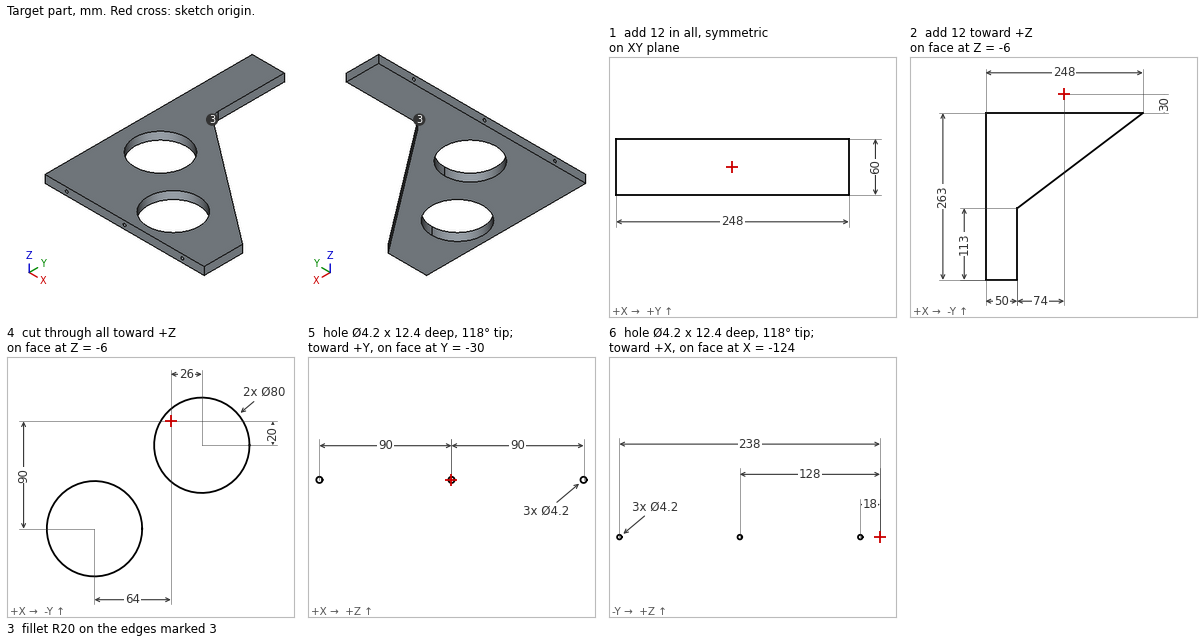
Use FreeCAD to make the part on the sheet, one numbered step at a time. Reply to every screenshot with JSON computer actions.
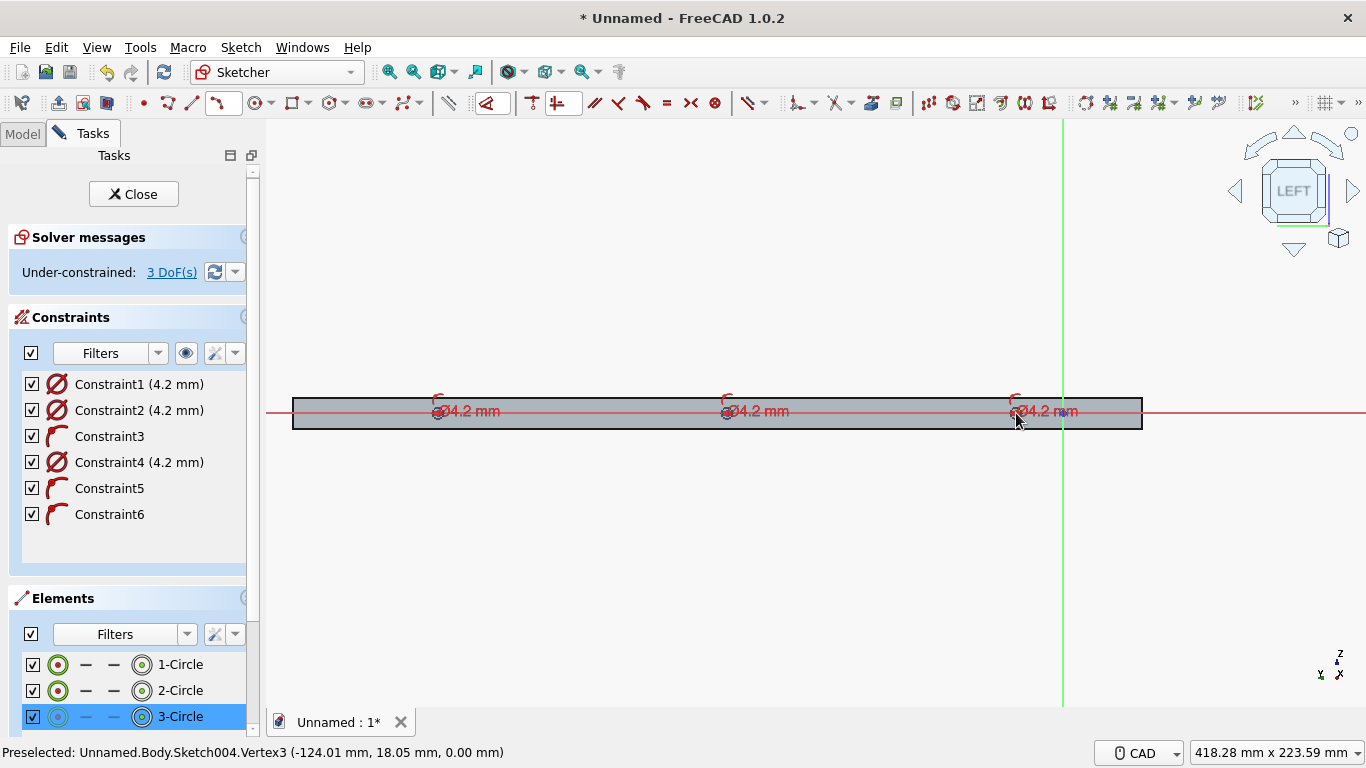
{"action": "key", "text": "l"}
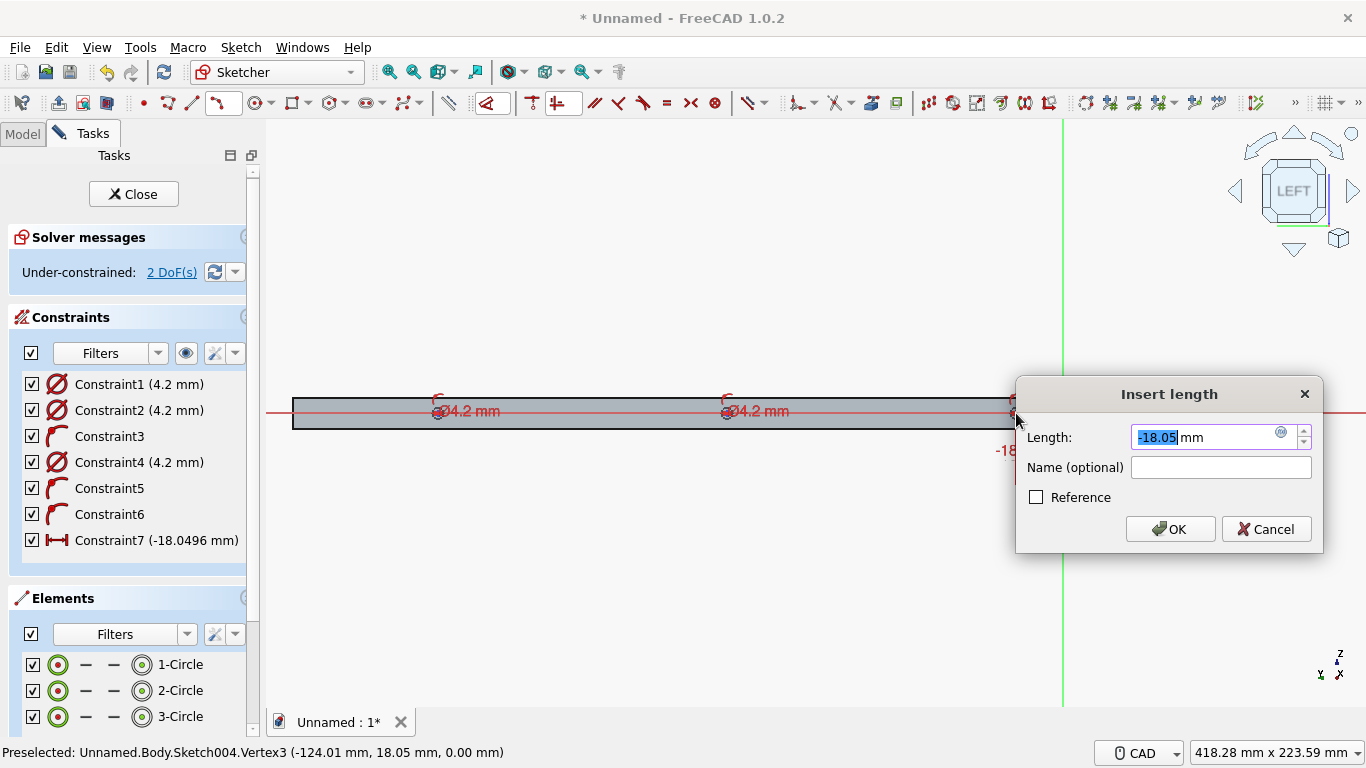
{"action": "type", "text": "-18"}
{"action": "key", "text": "Return"}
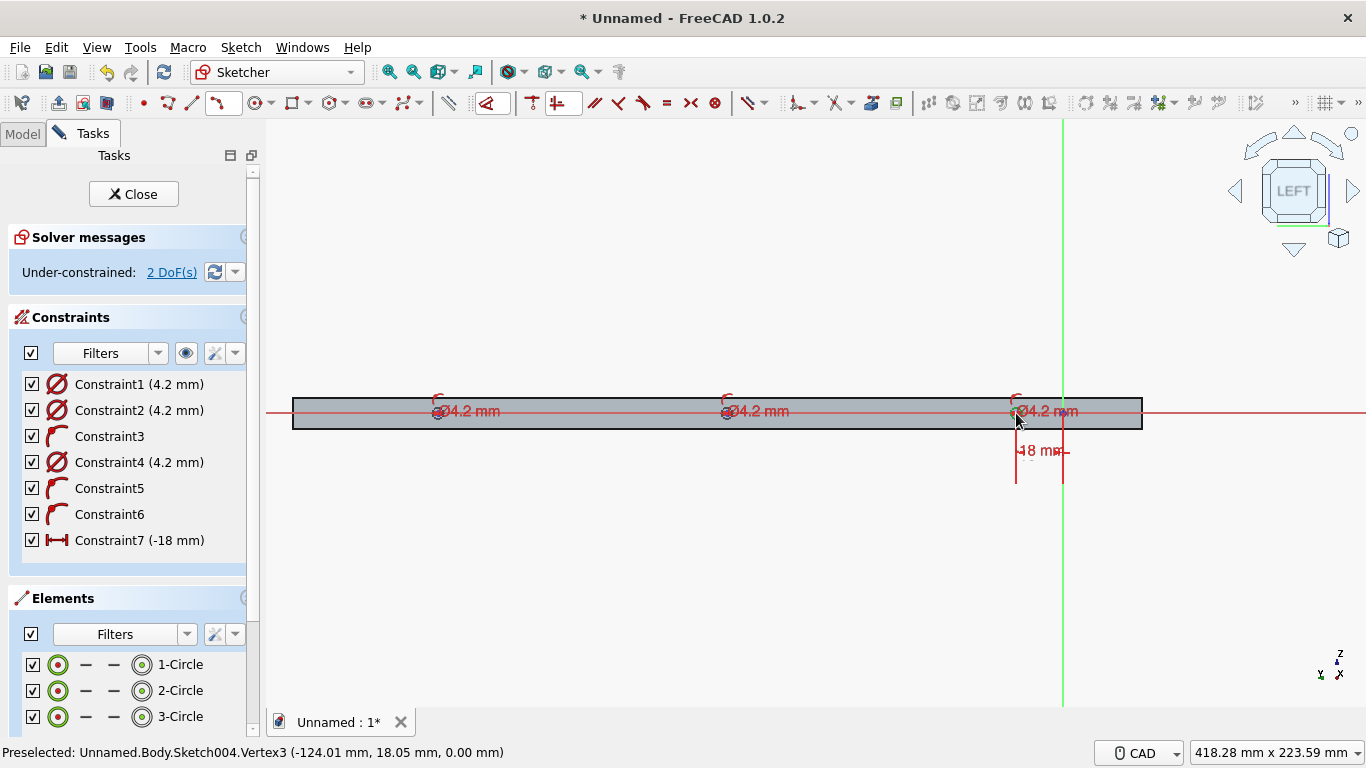
{"action": "left_click", "coordinate": [438, 413]}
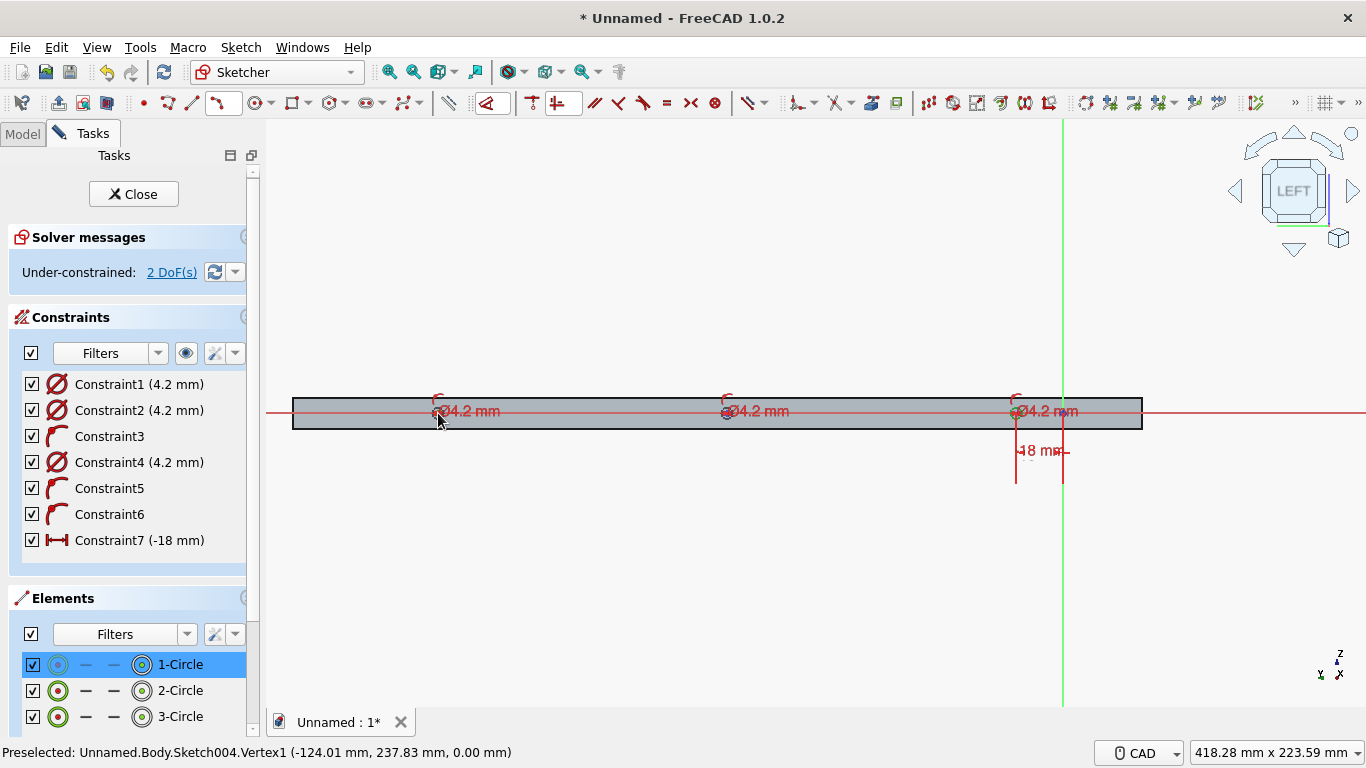
{"action": "key", "text": "l"}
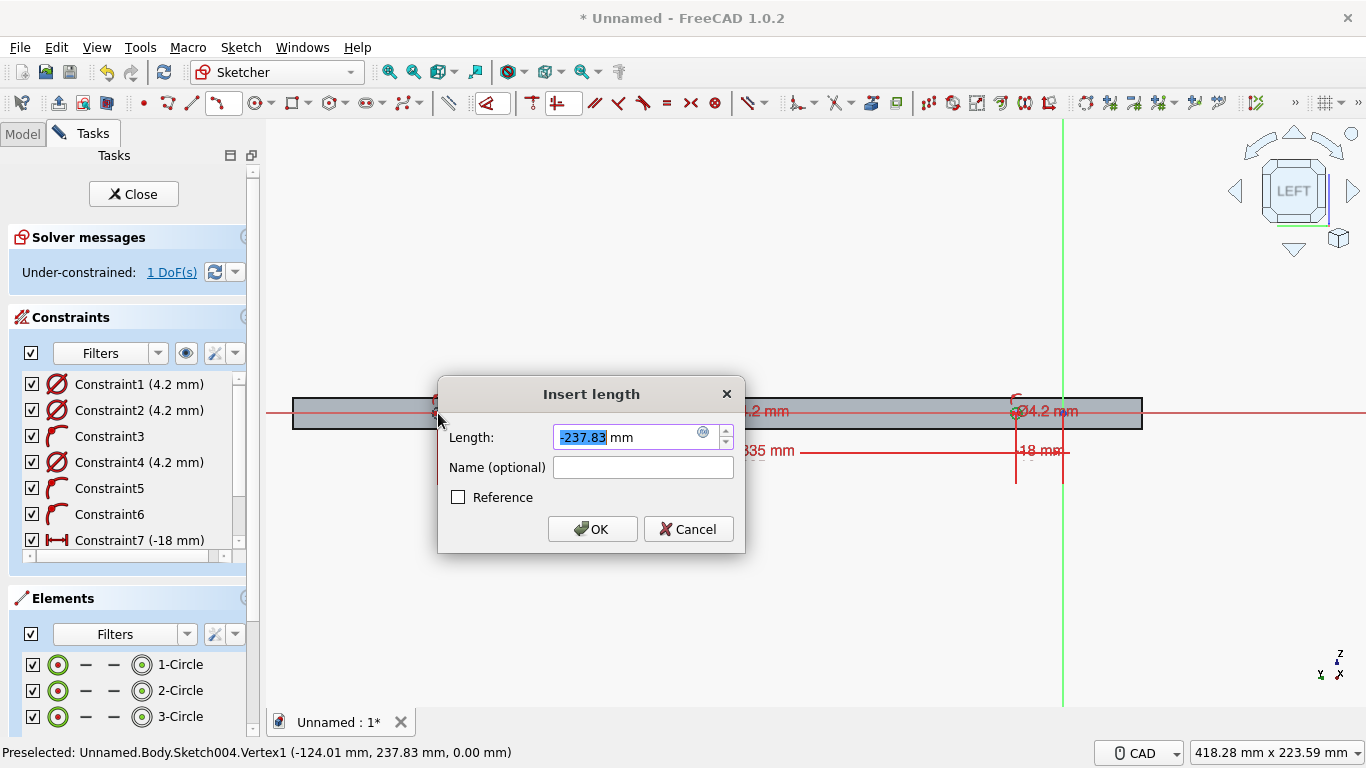
{"action": "type", "text": "-238"}
{"action": "key", "text": "Return"}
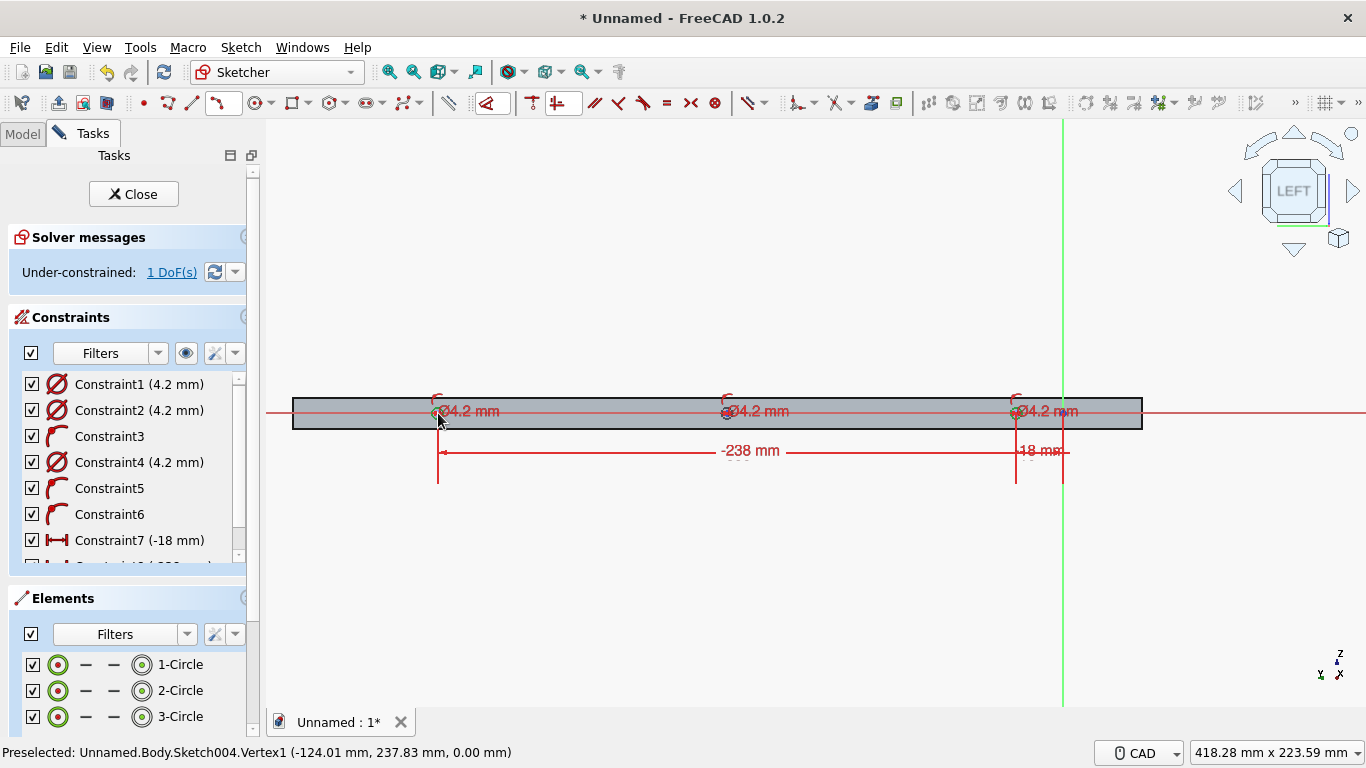
{"action": "left_click", "coordinate": [727, 413]}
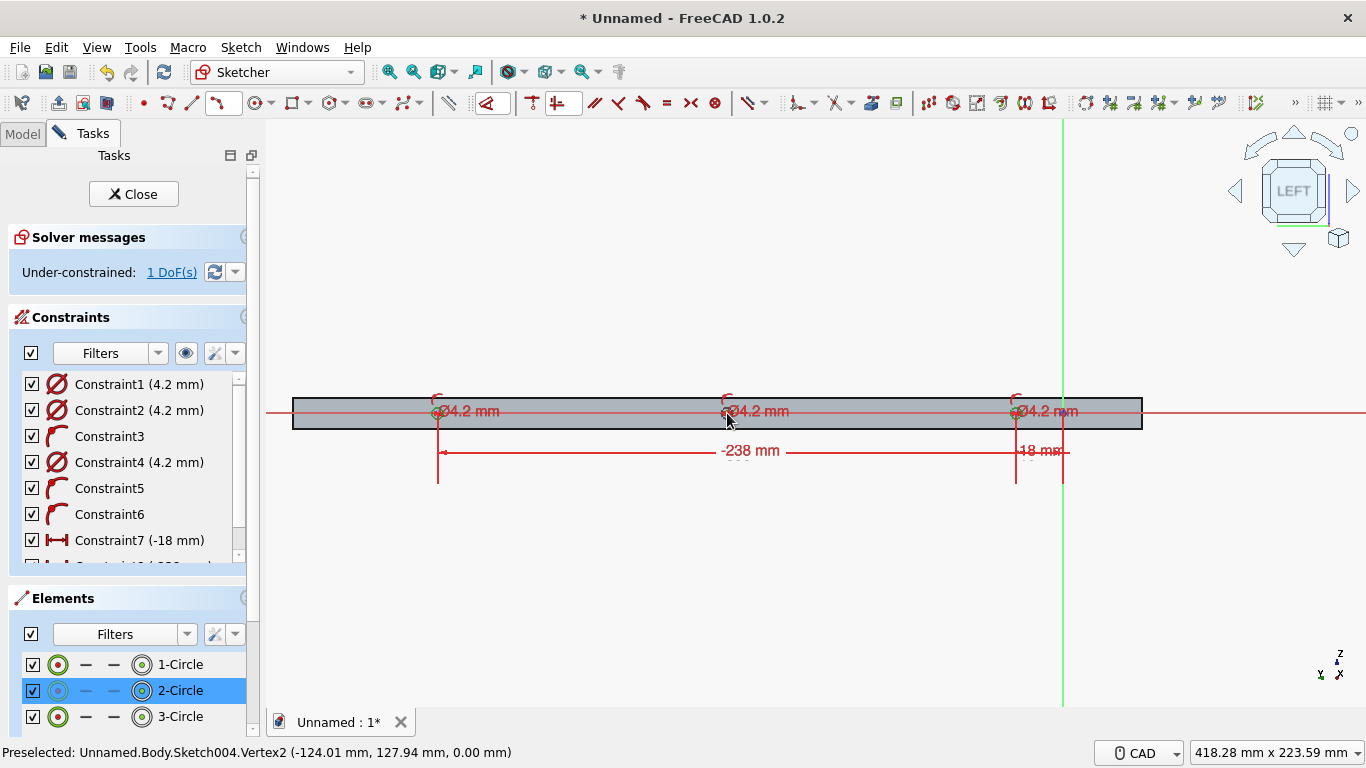
{"action": "key", "text": "l"}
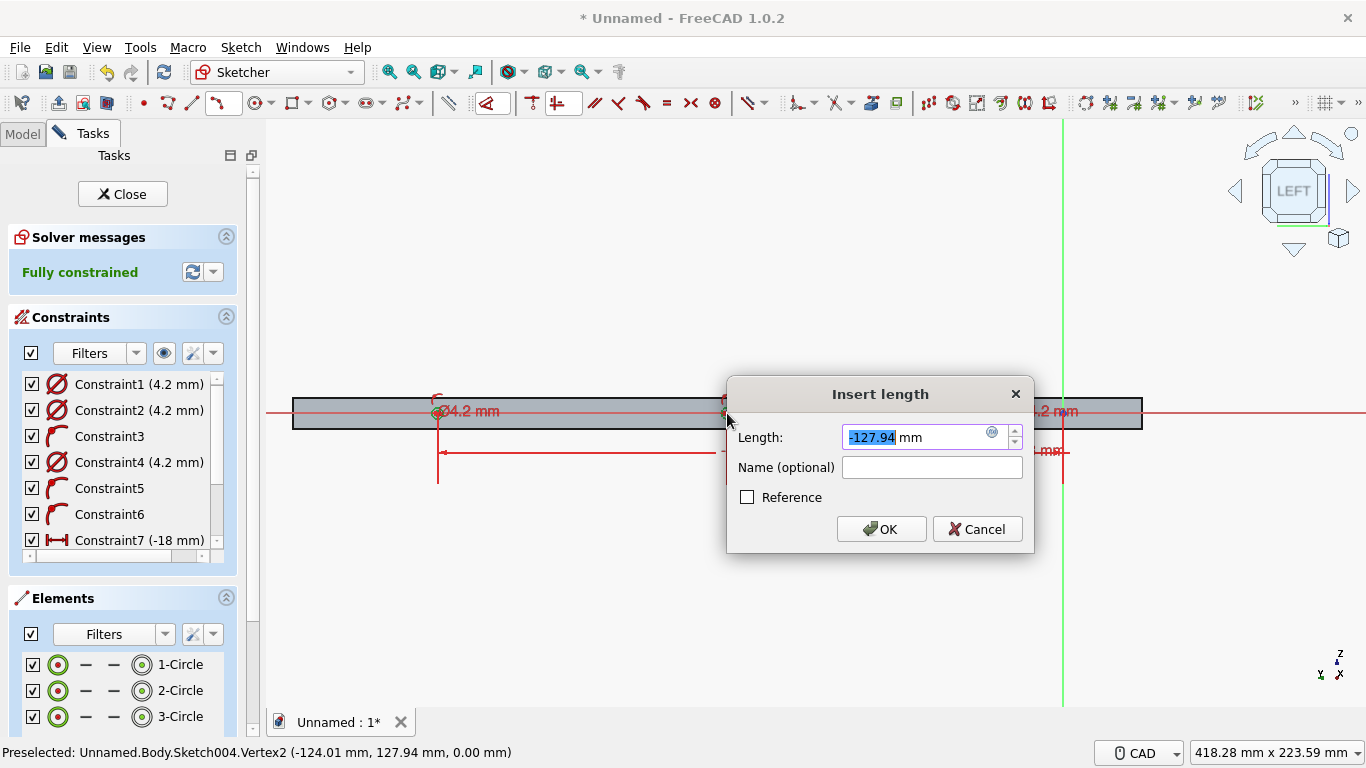
{"action": "type", "text": "-128"}
{"action": "key", "text": "Return"}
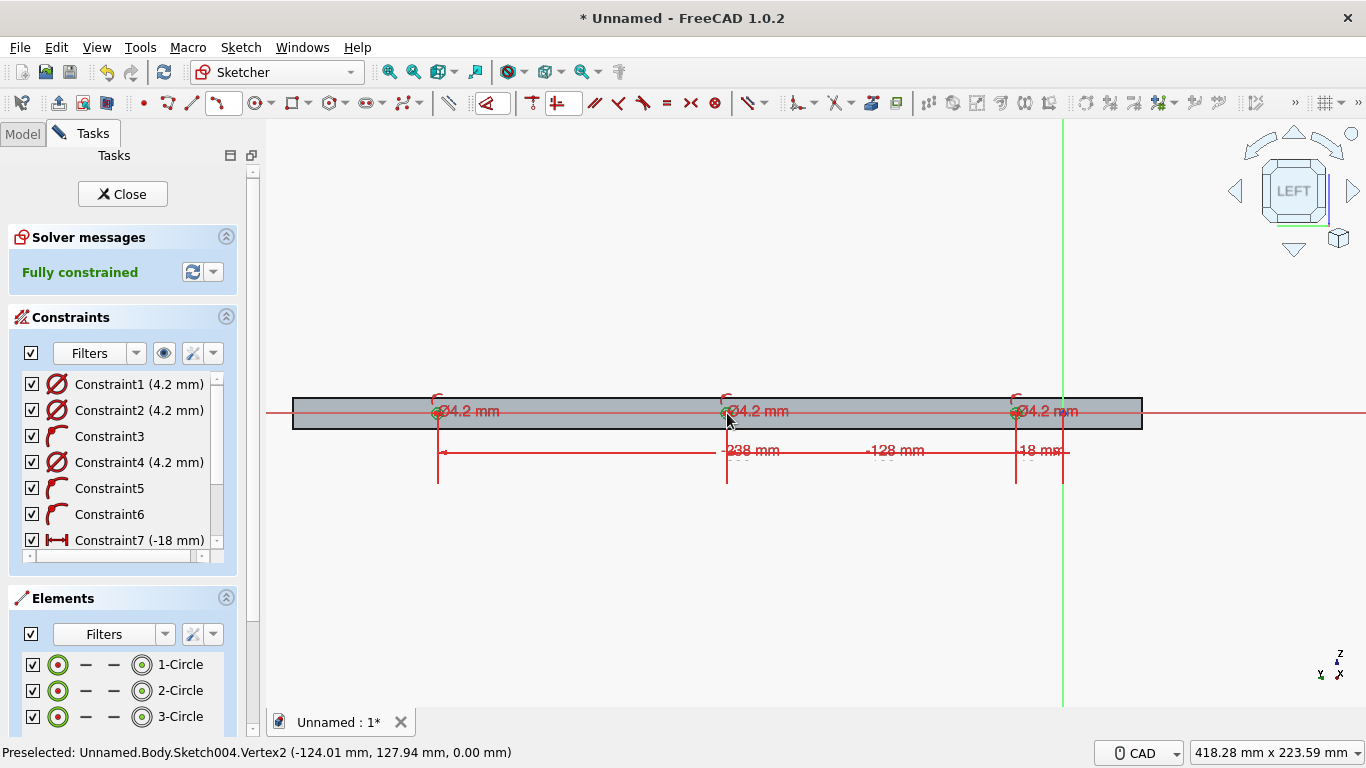
{"action": "left_click", "coordinate": [123, 194]}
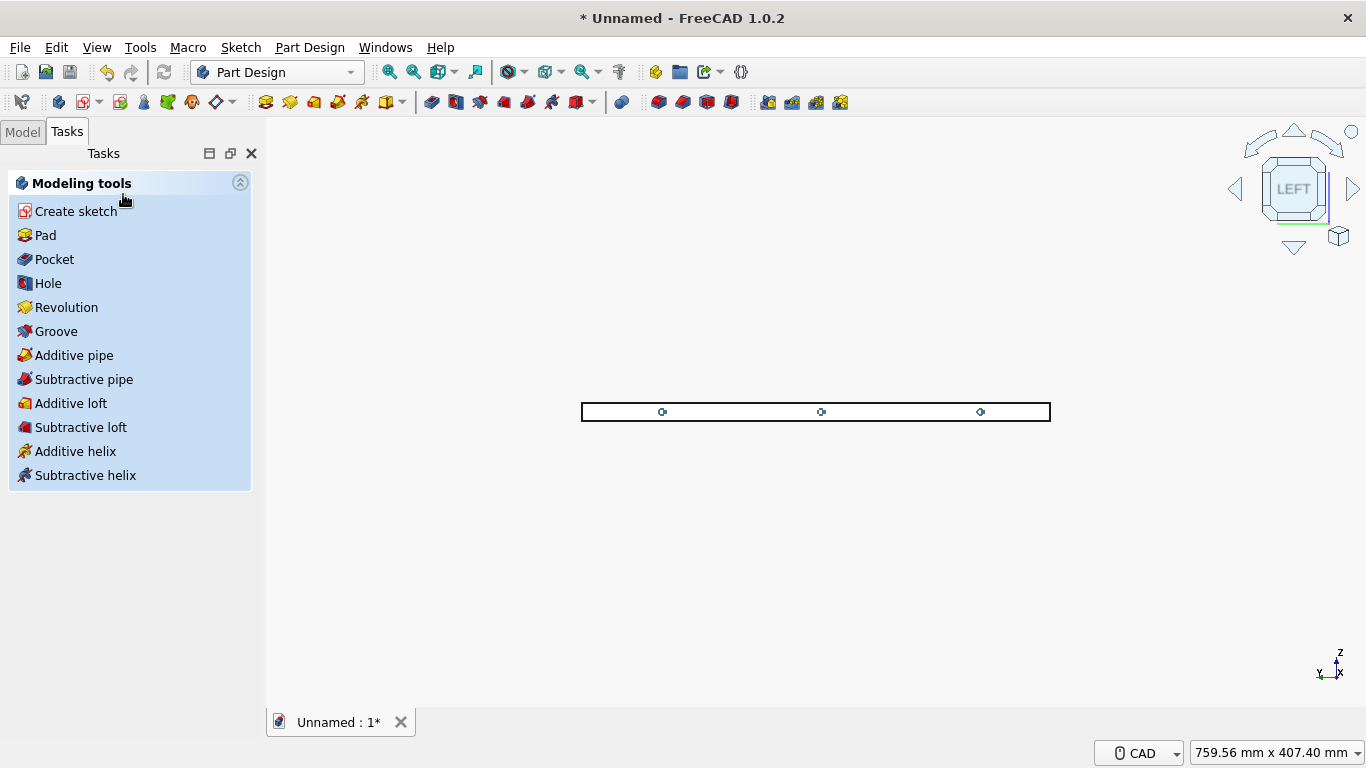
{"action": "left_click", "coordinate": [456, 102]}